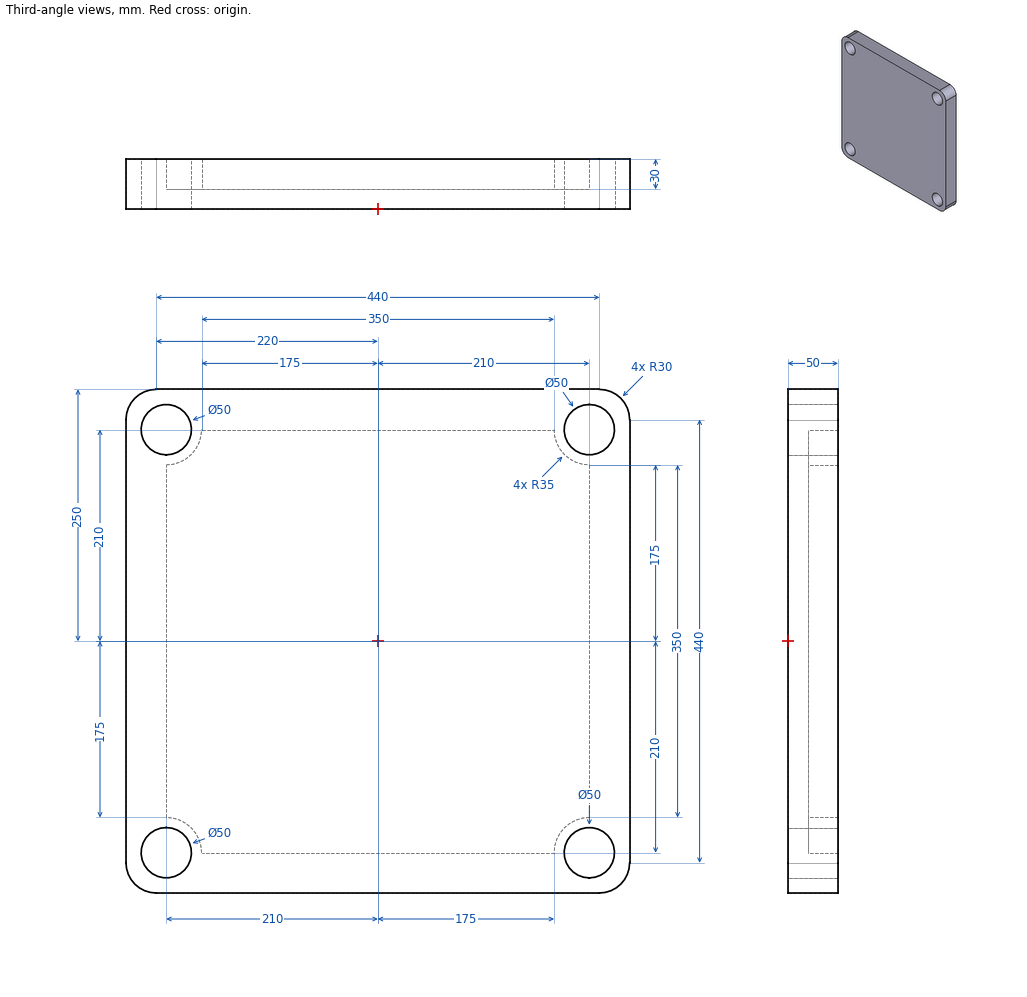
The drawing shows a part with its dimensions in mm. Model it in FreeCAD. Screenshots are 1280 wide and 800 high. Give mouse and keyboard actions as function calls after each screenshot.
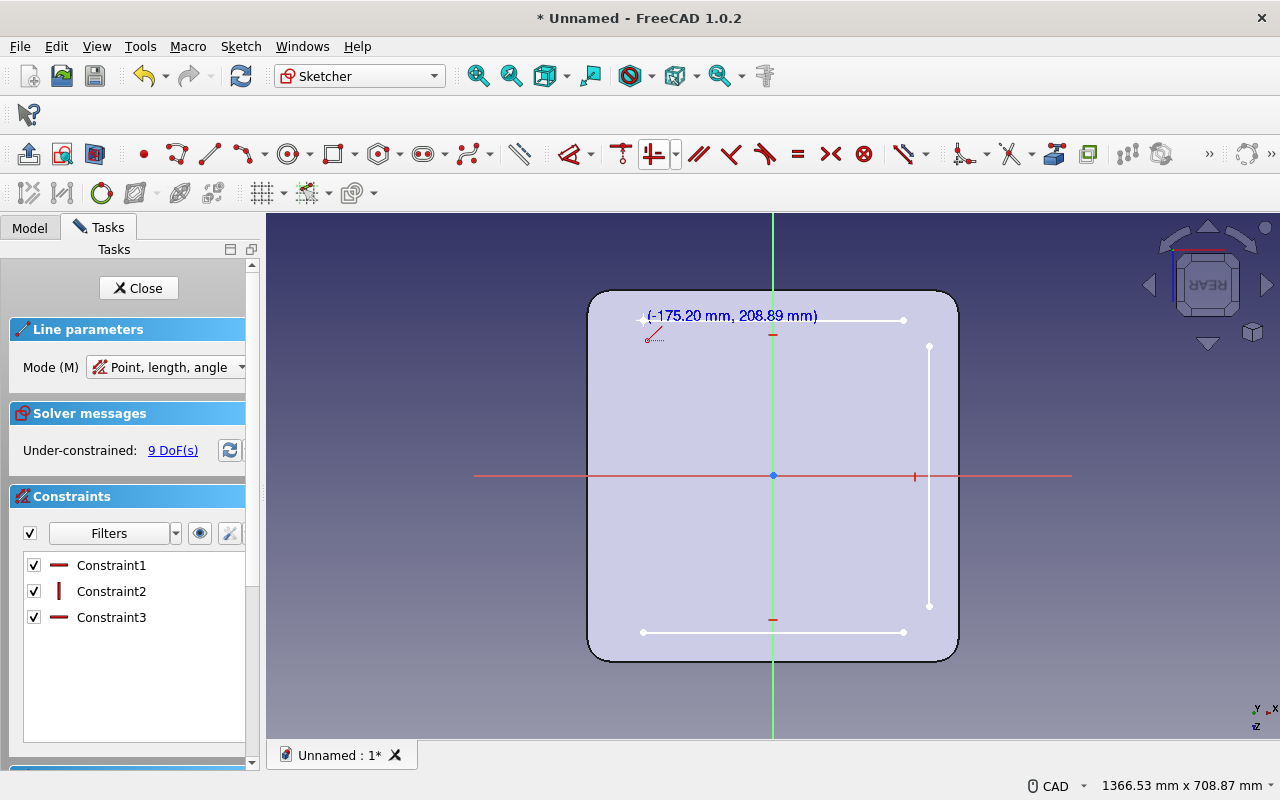
click(617, 346)
click(617, 606)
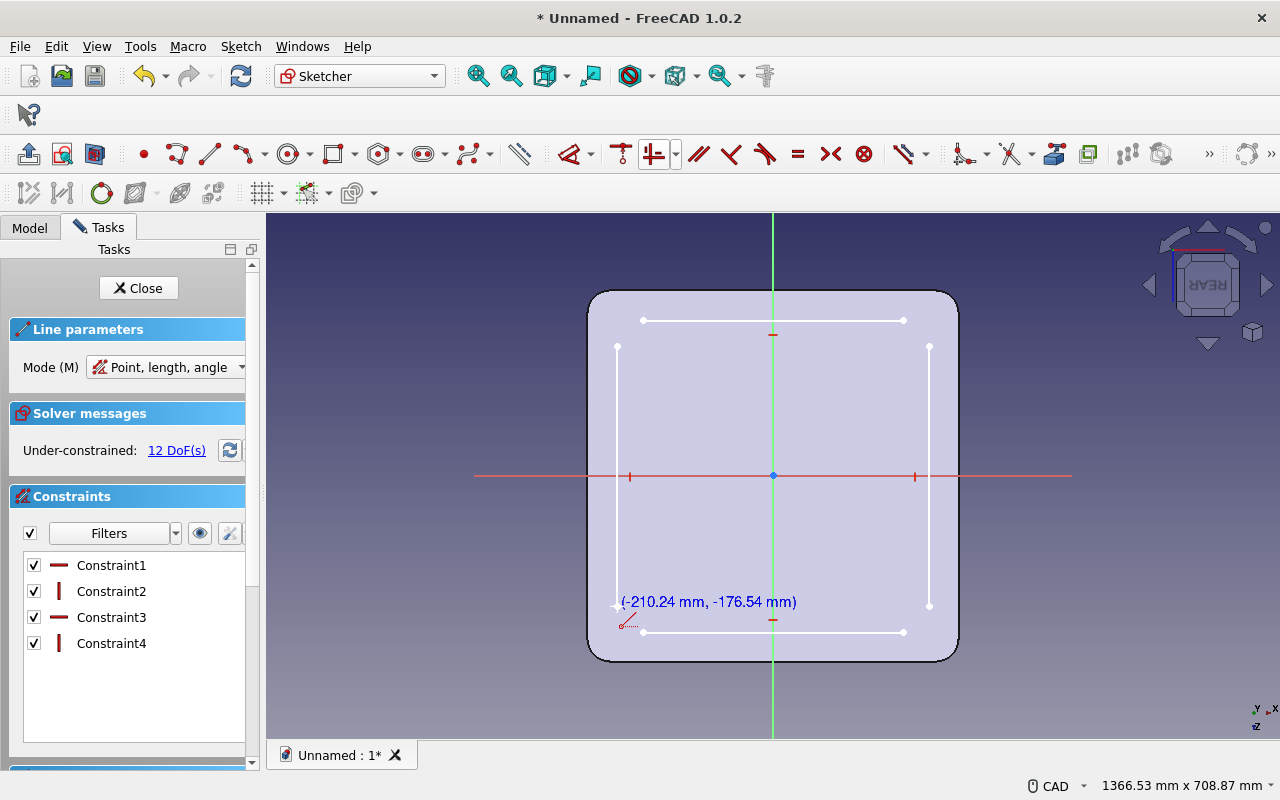
click(242, 154)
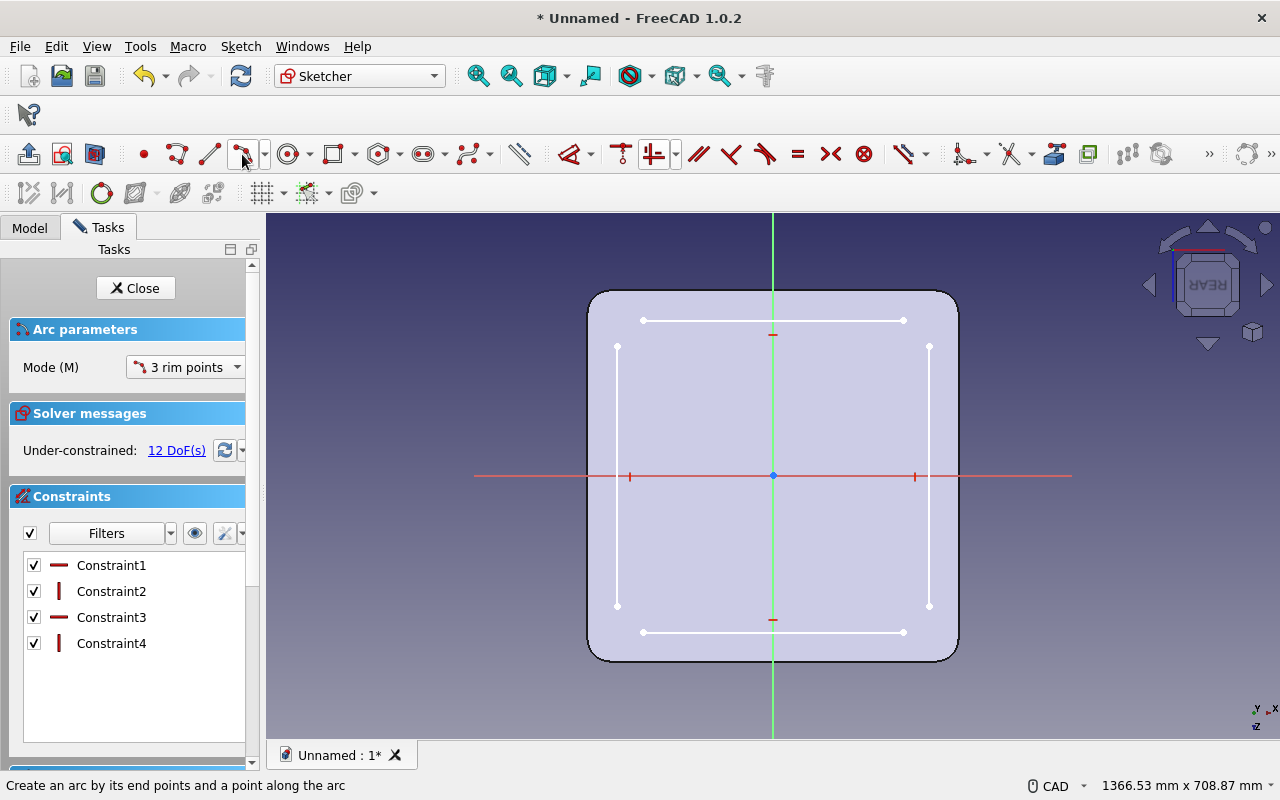
click(903, 633)
click(929, 607)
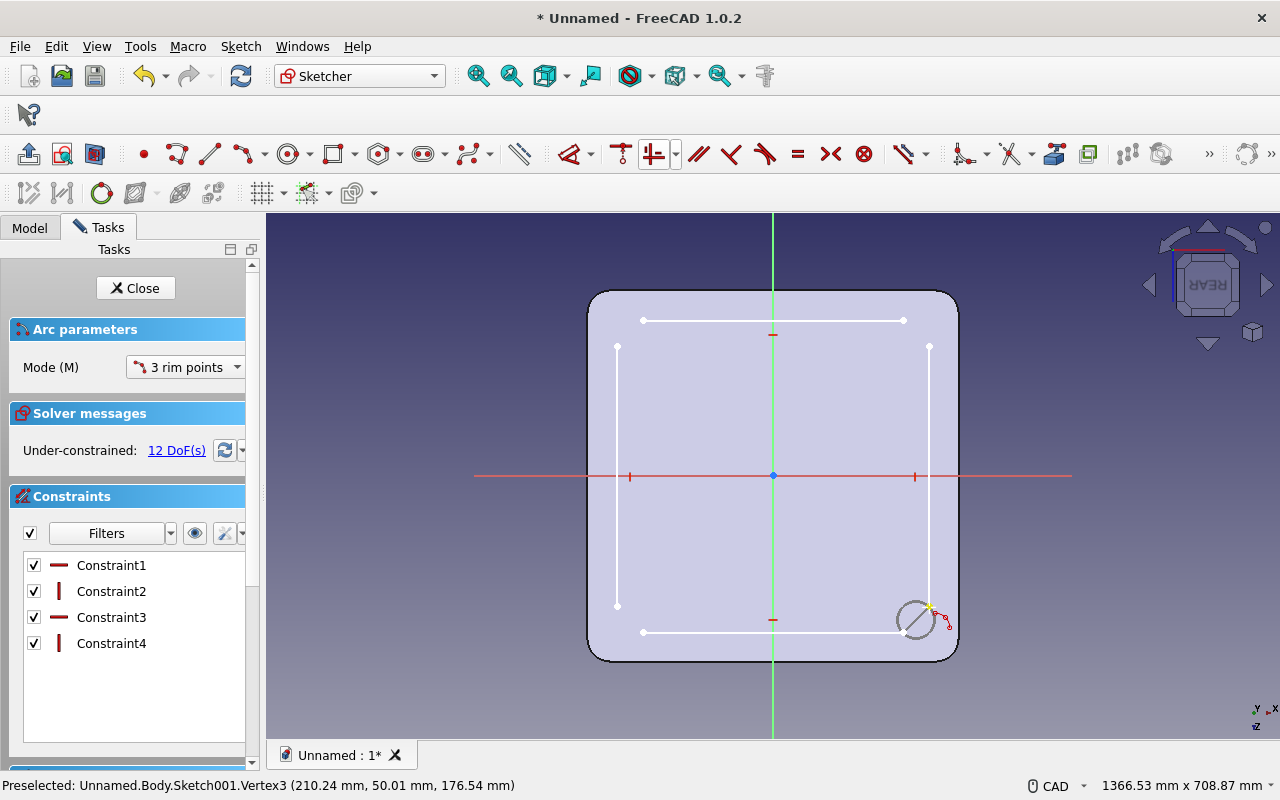
scroll(910, 613, up, 4)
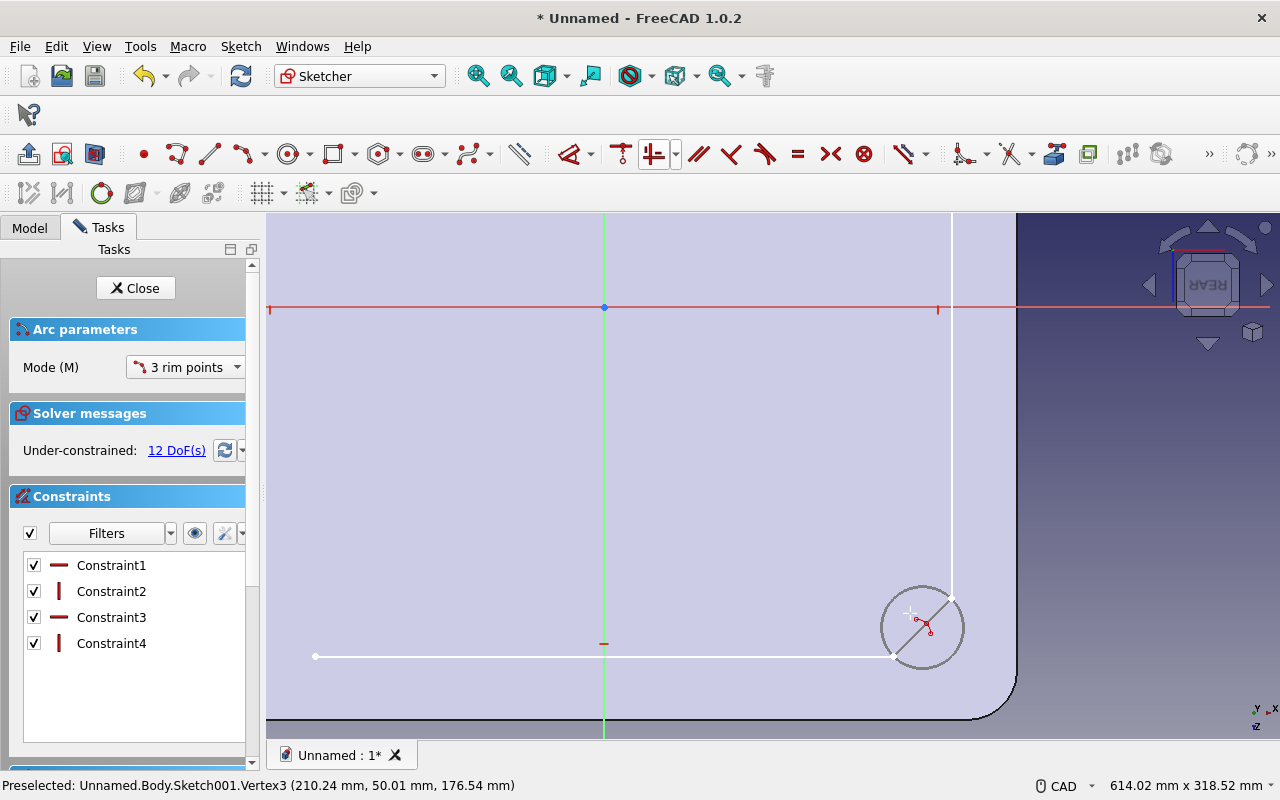
click(910, 613)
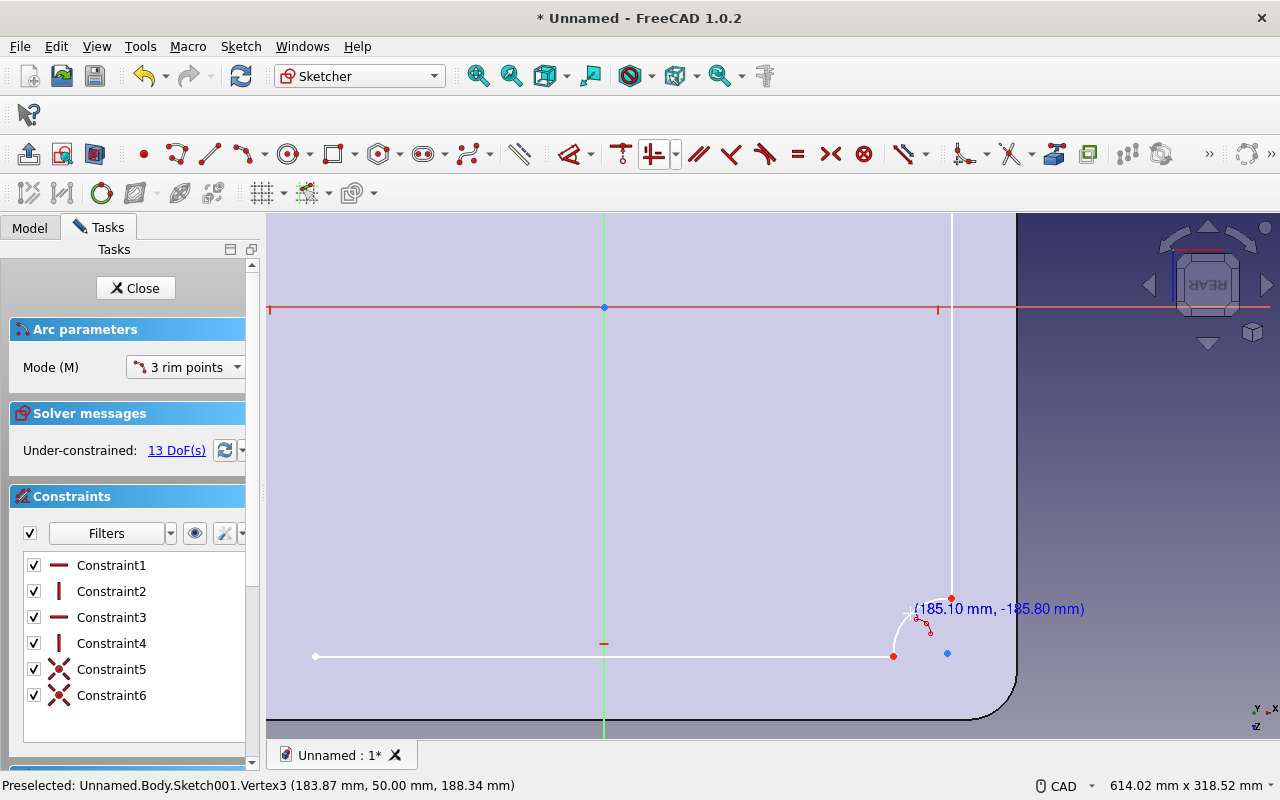
scroll(786, 614, down, 4)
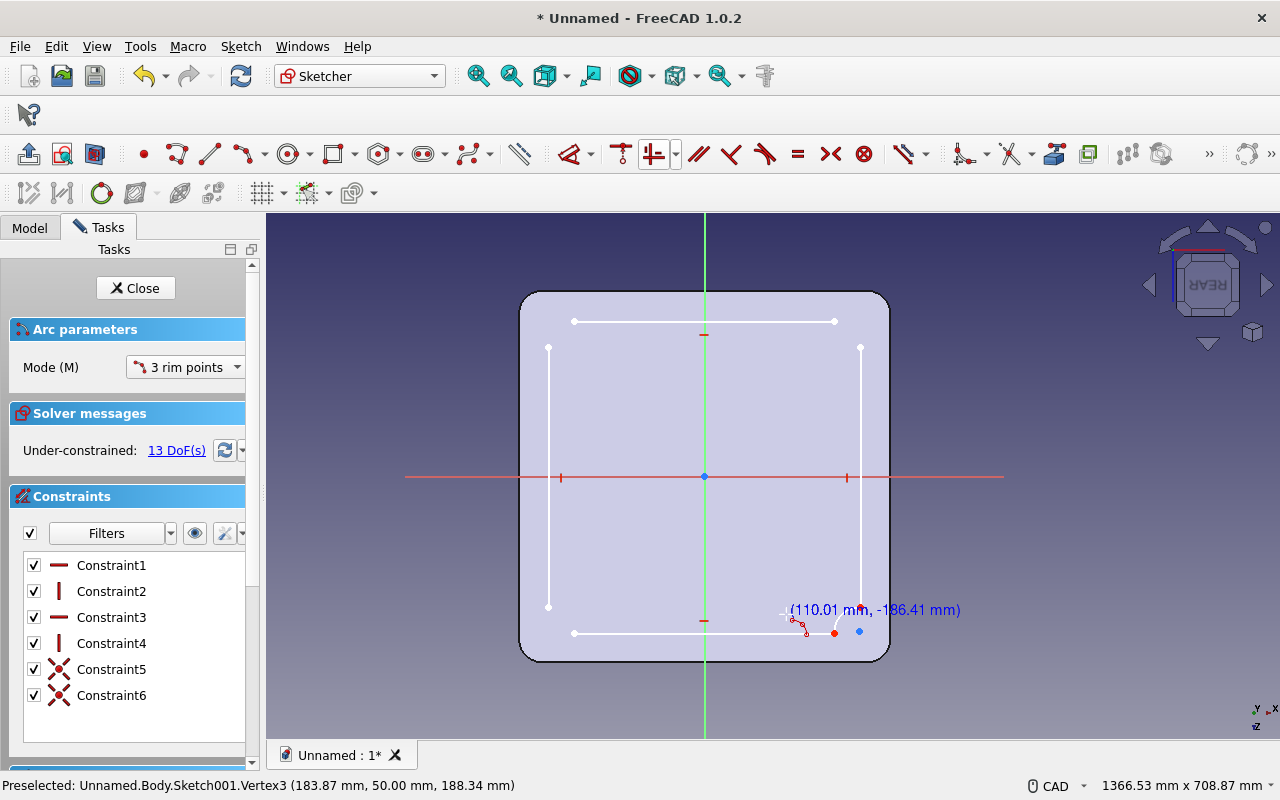
click(861, 348)
click(835, 322)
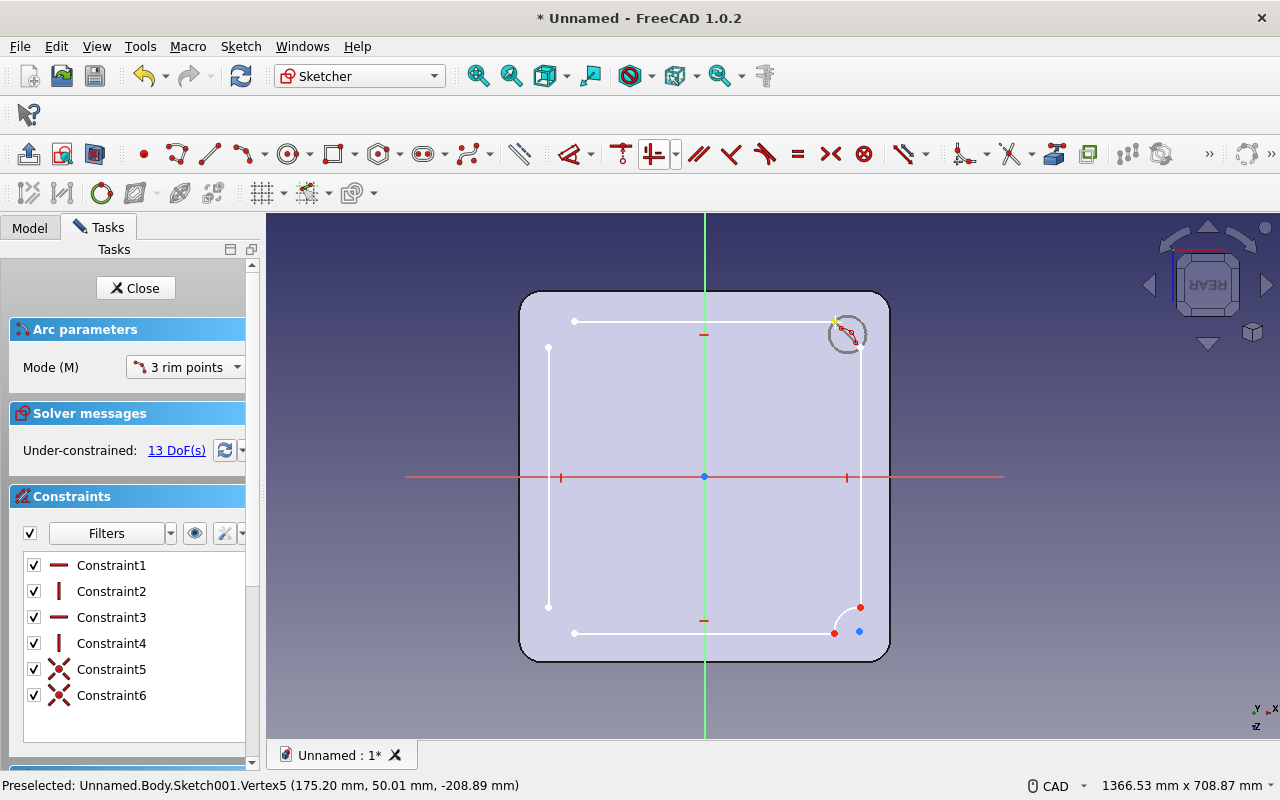
scroll(842, 339, up, 4)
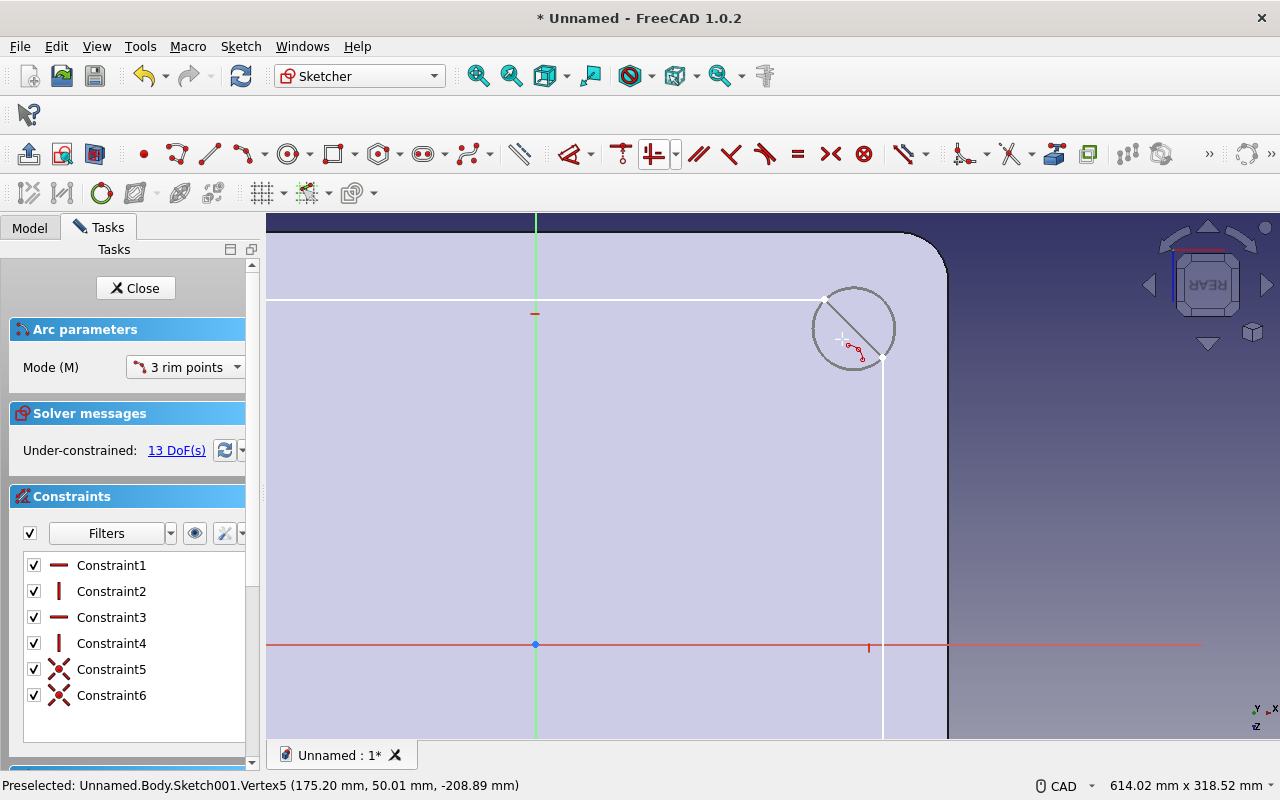
click(842, 339)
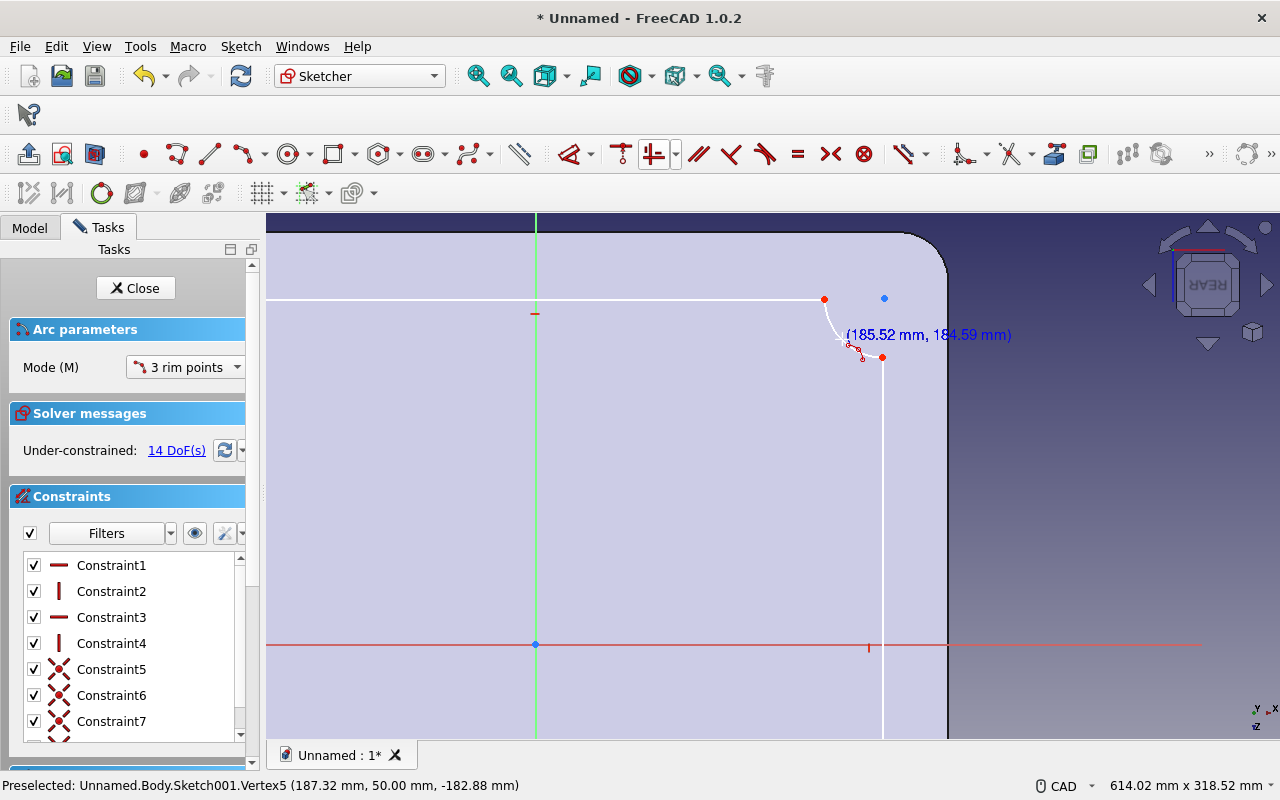
scroll(842, 338, down, 4)